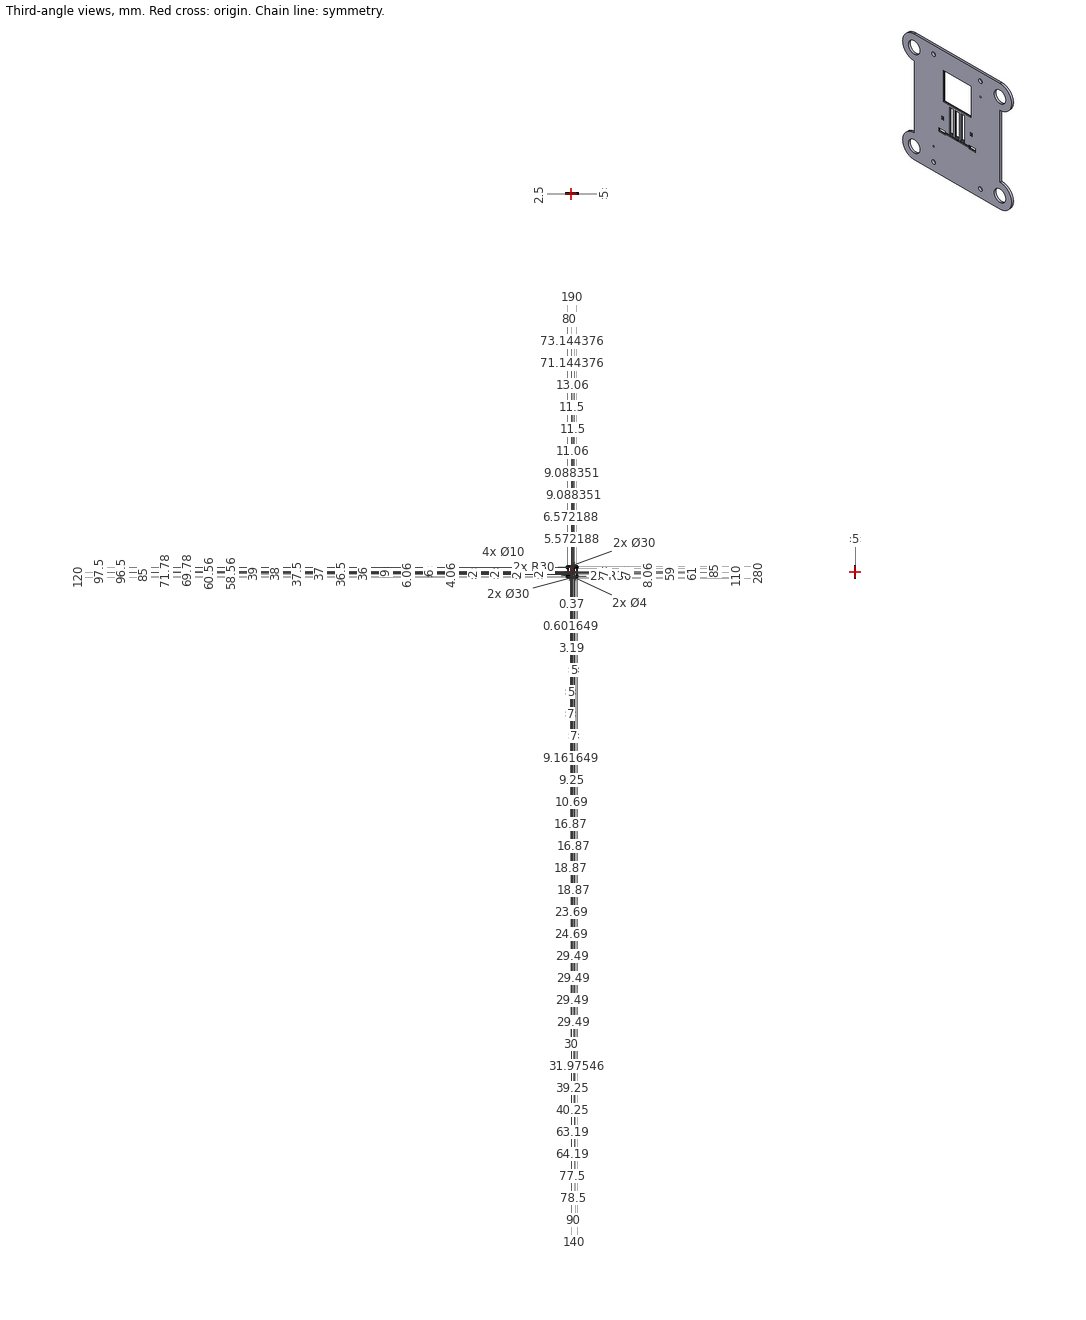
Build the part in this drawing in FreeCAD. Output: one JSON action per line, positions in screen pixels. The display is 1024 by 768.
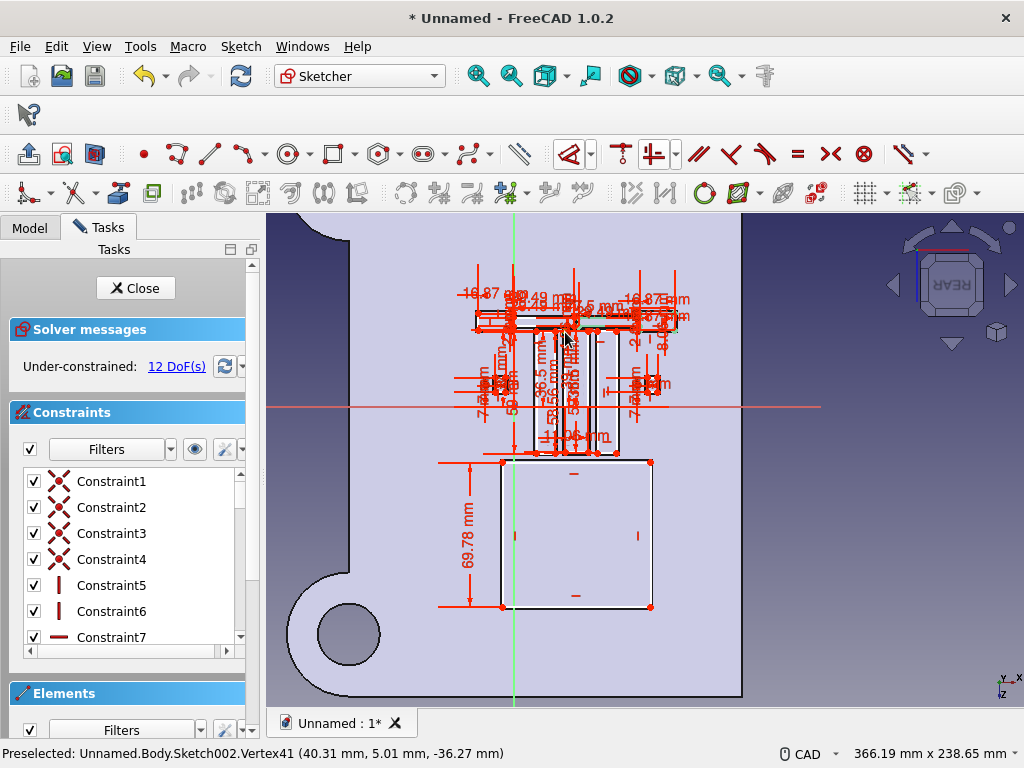
{"action": "left_click", "coordinate": [503, 607]}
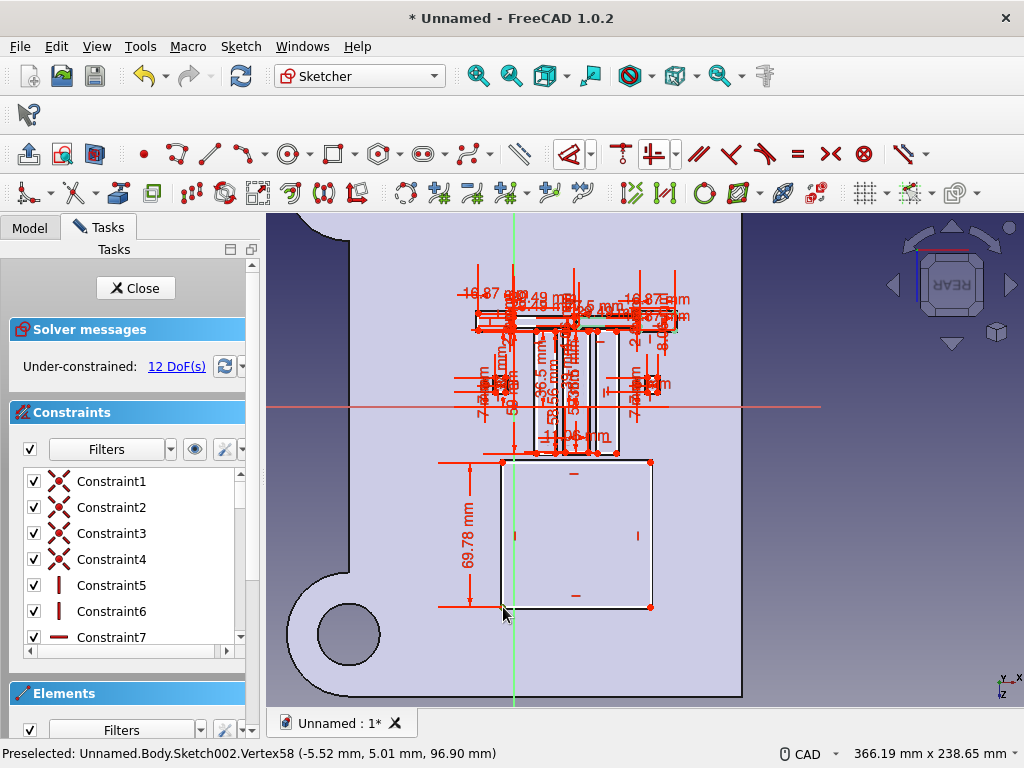
{"action": "key", "text": "i"}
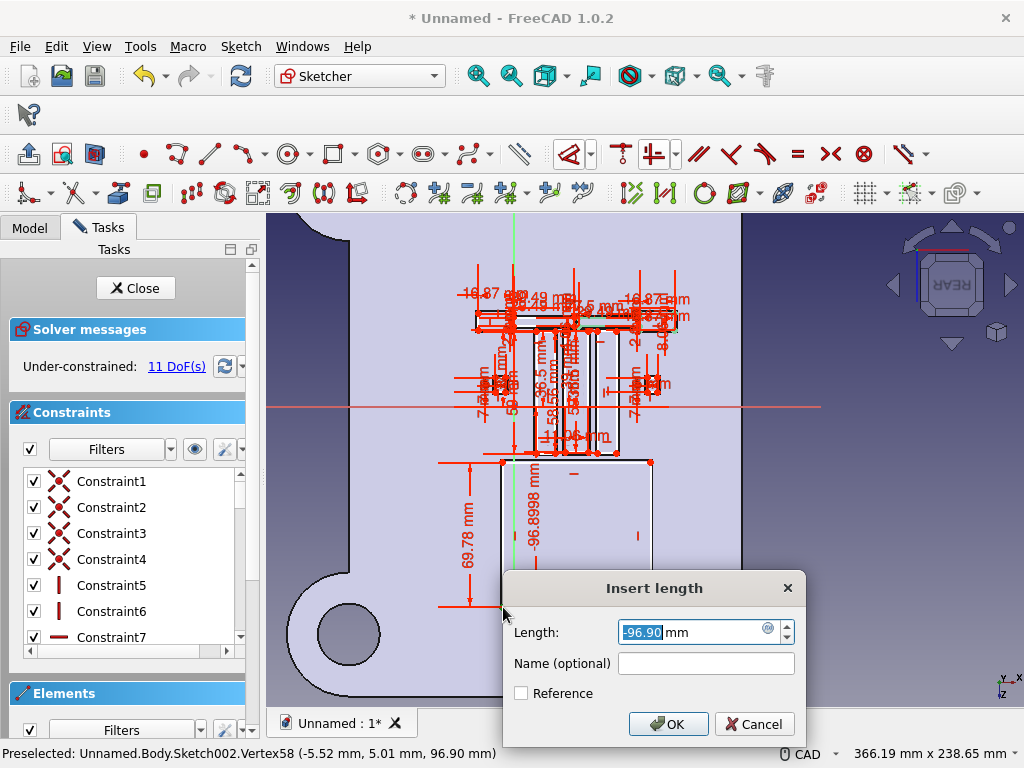
{"action": "type", "text": "-96.5"}
{"action": "key", "text": "Return"}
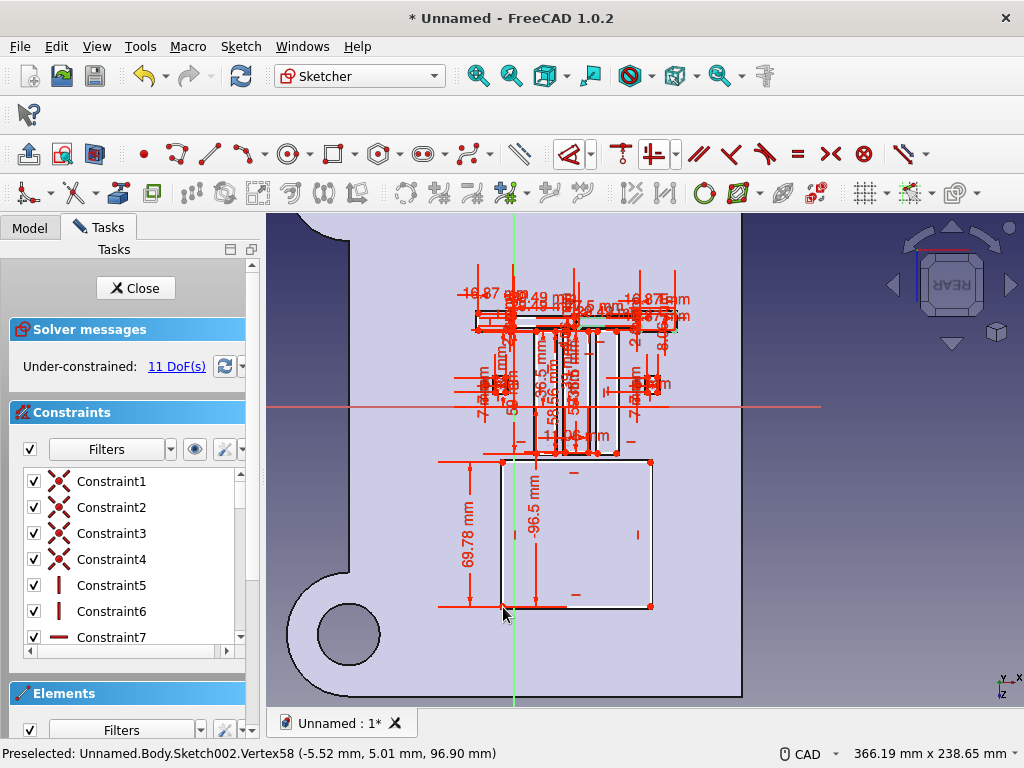
{"action": "left_click", "coordinate": [537, 332]}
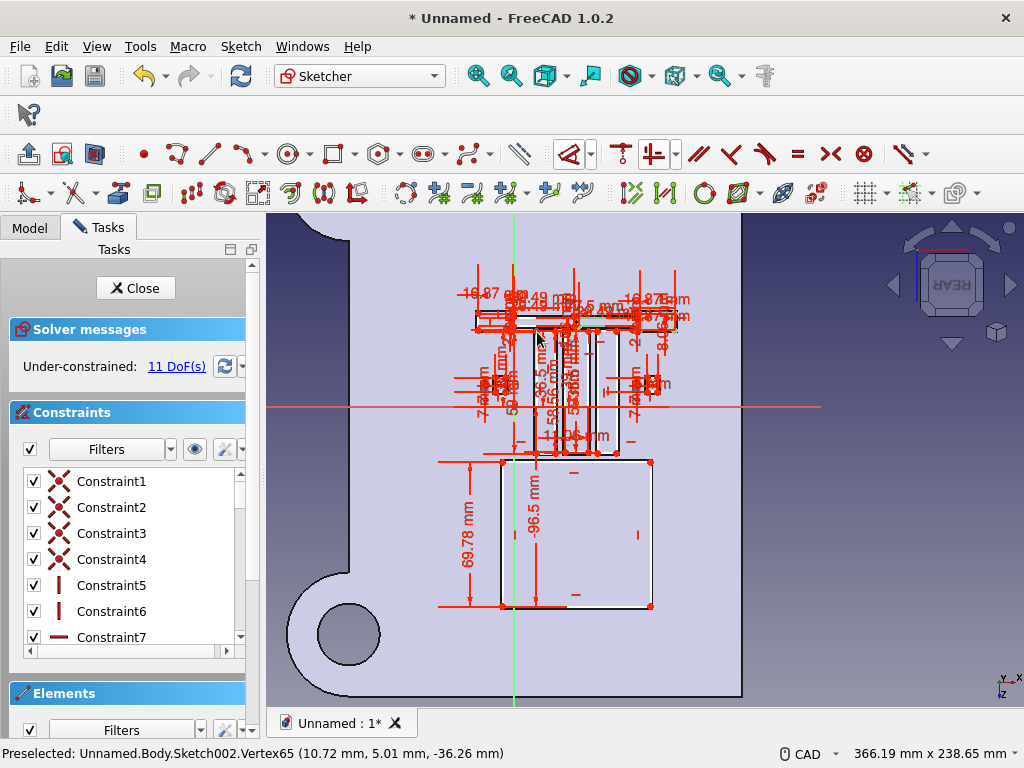
{"action": "key", "text": "i"}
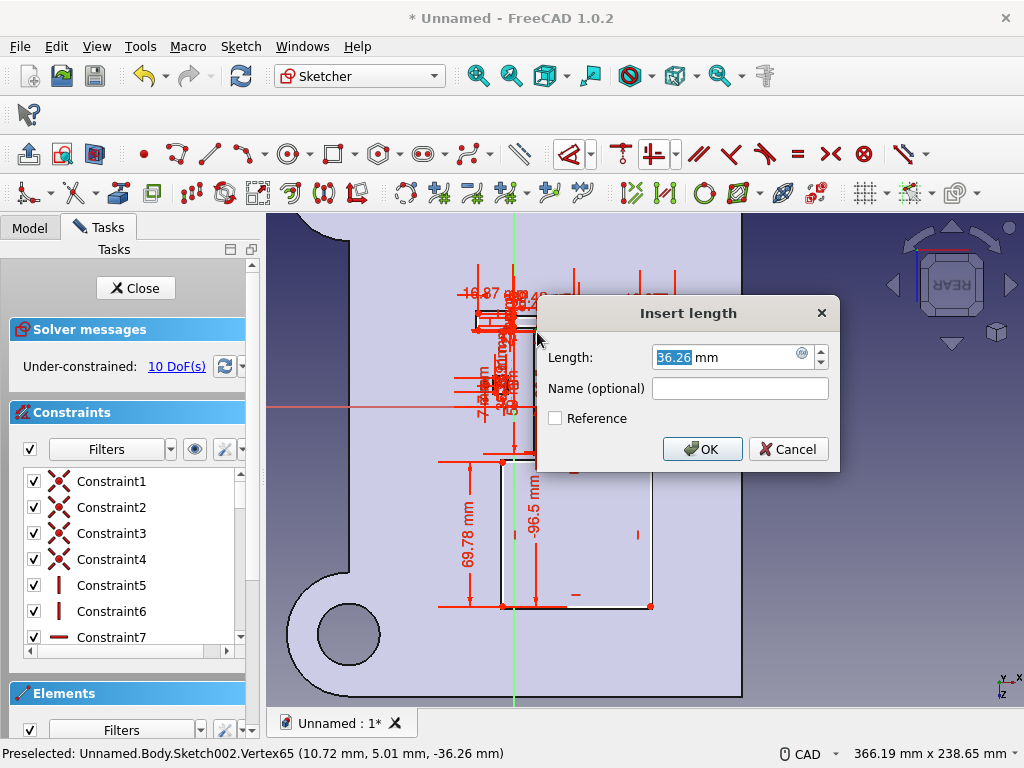
{"action": "type", "text": "36.5"}
{"action": "key", "text": "Return"}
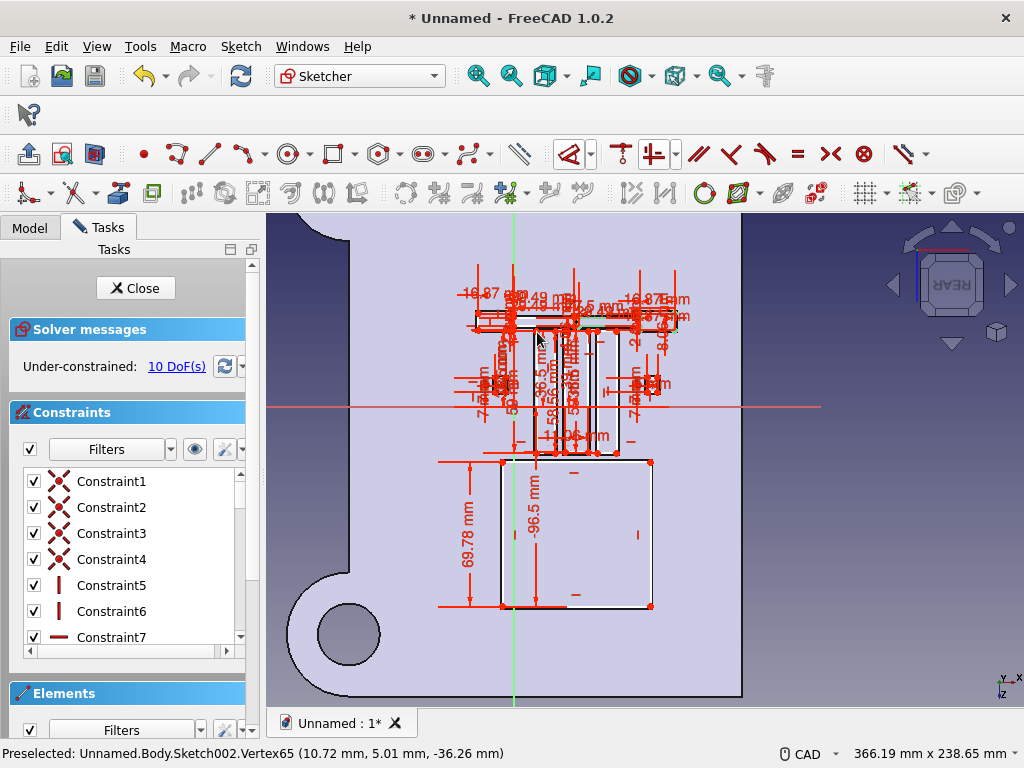
{"action": "scroll", "coordinate": [565, 331], "scroll_direction": "up", "scroll_amount": 2}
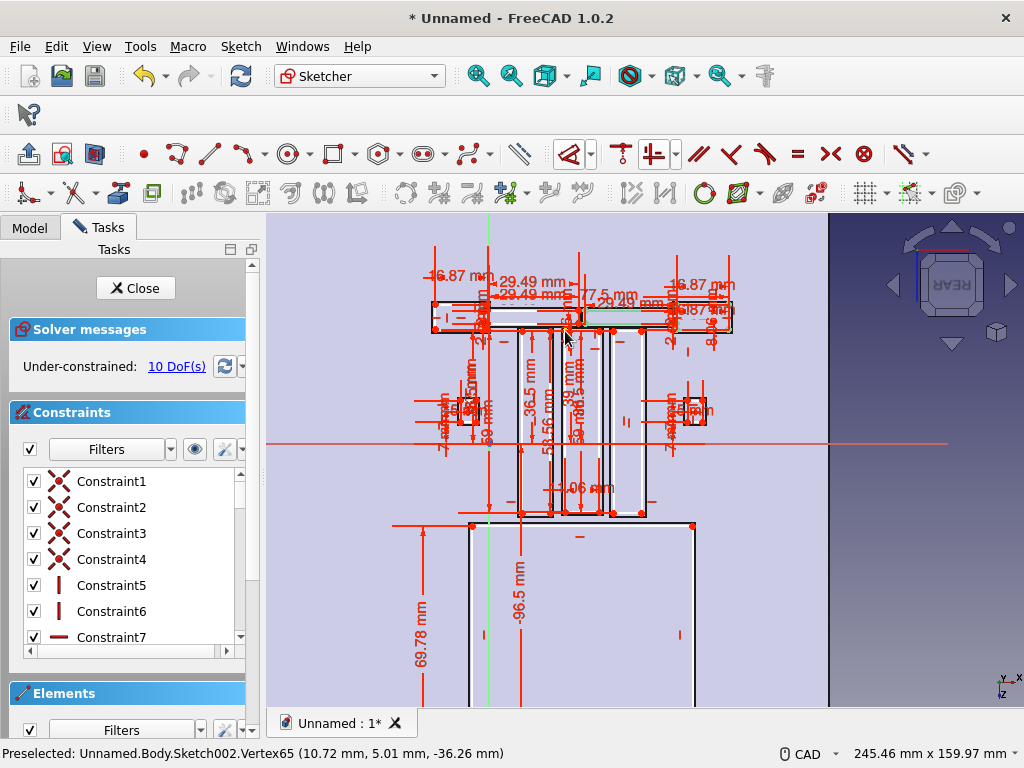
{"action": "left_click", "coordinate": [565, 331]}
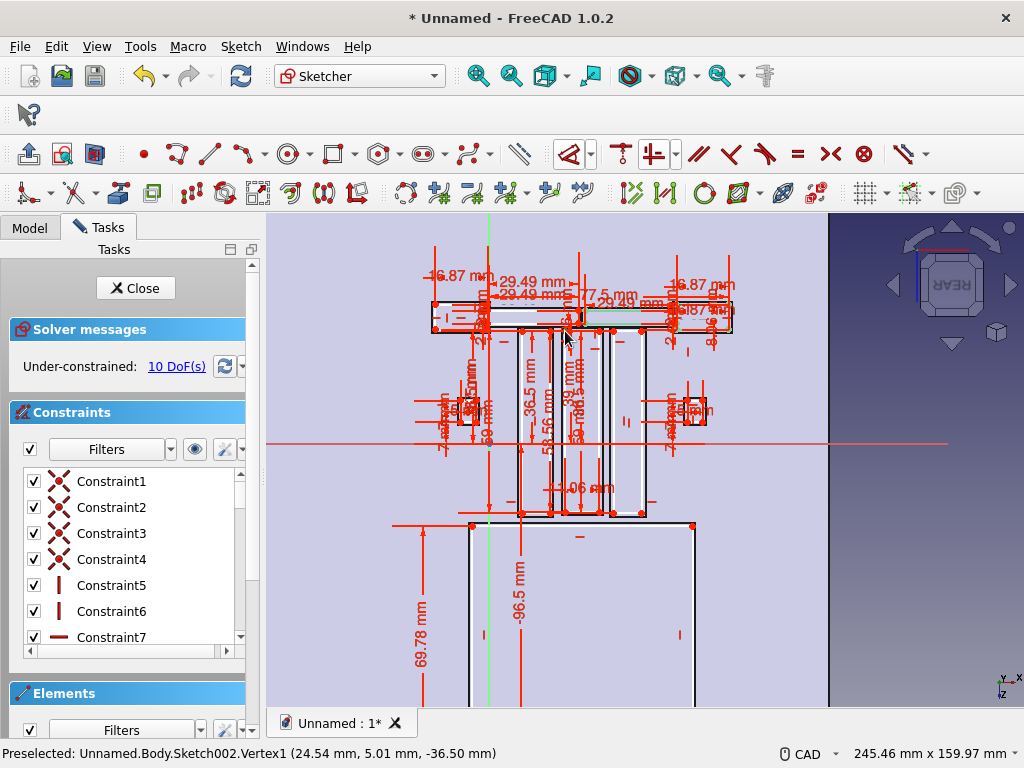
{"action": "key", "text": "l"}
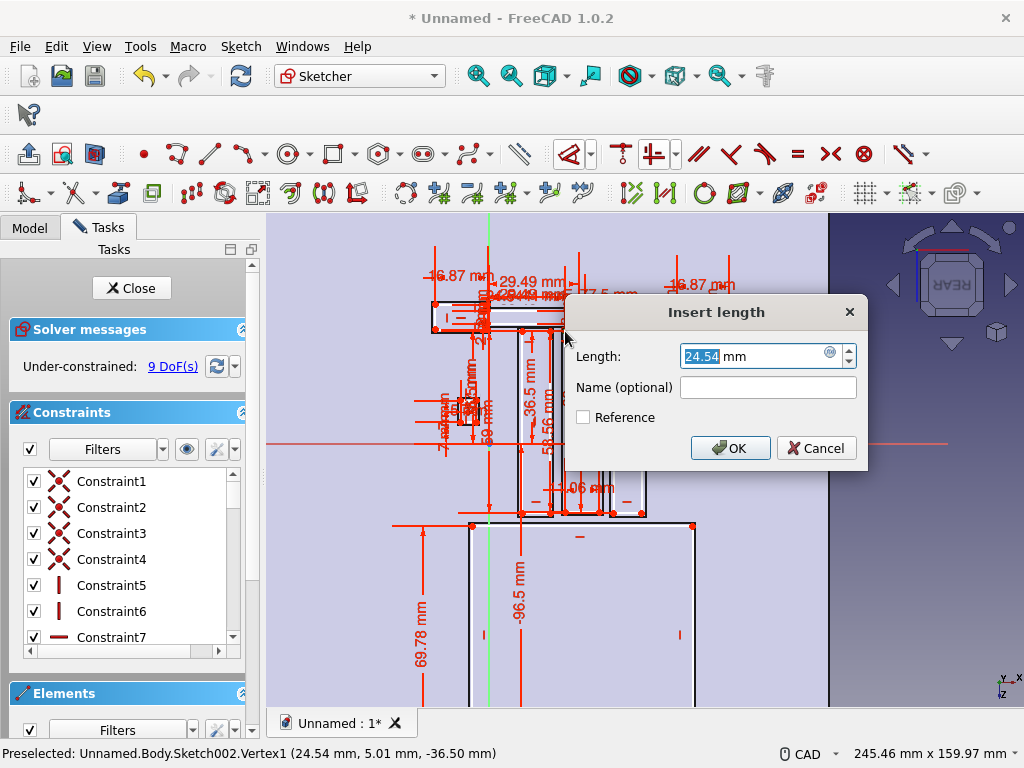
{"action": "type", "text": "24.69"}
{"action": "key", "text": "Return"}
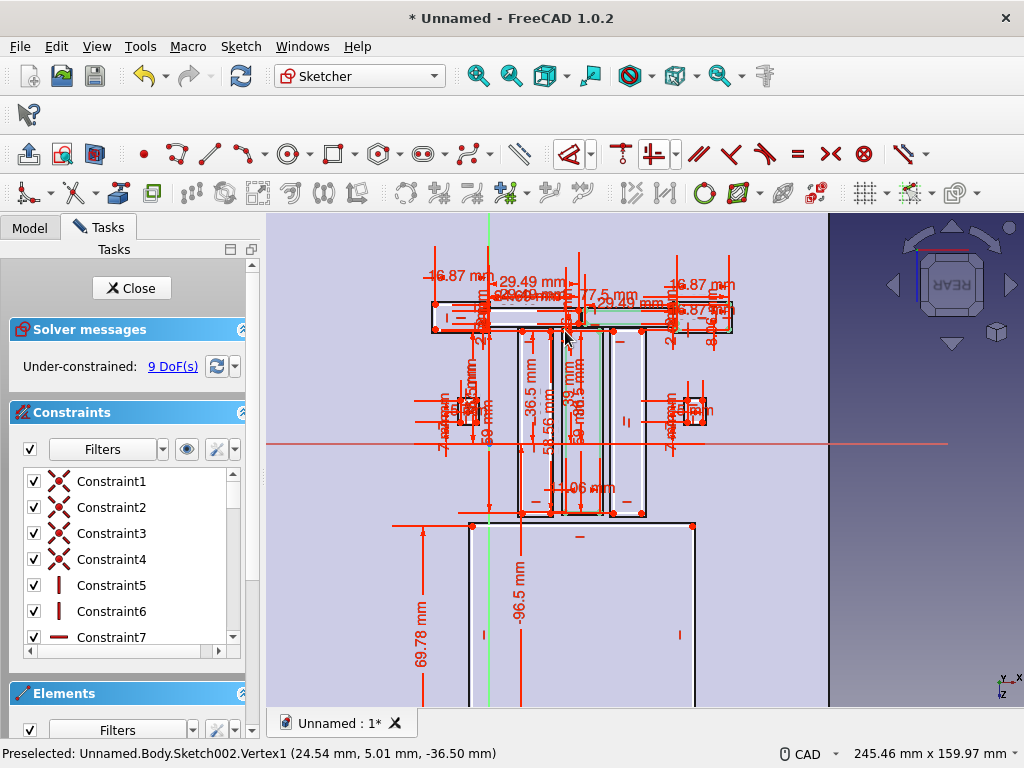
{"action": "left_click", "coordinate": [614, 331]}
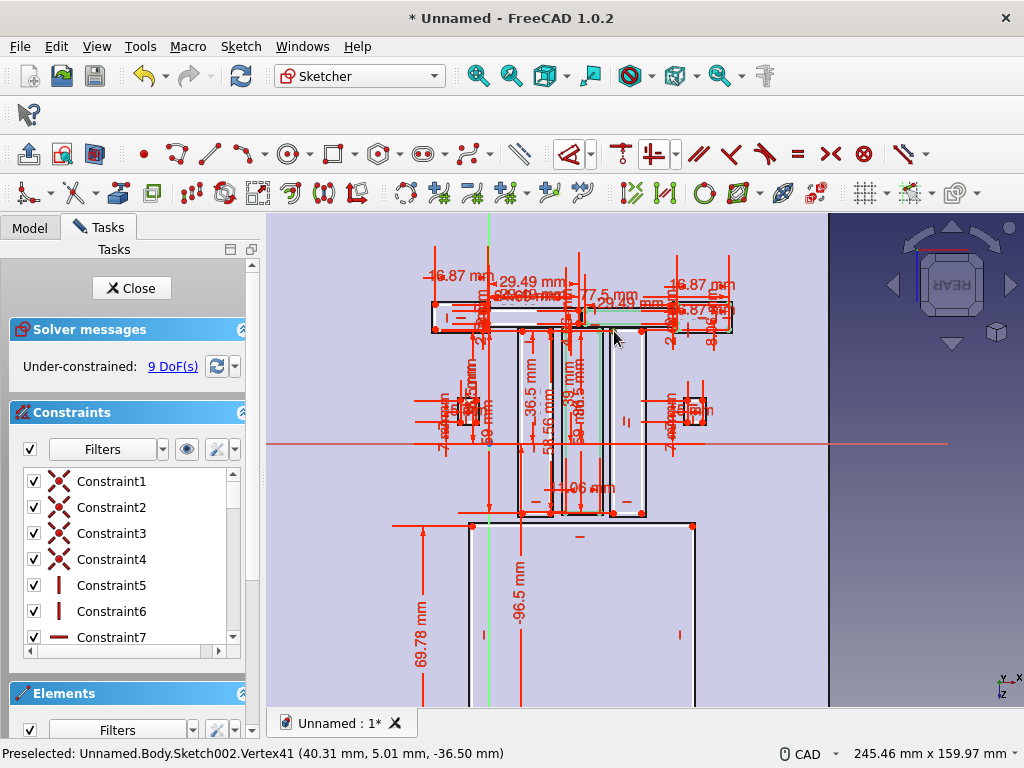
{"action": "key", "text": "l"}